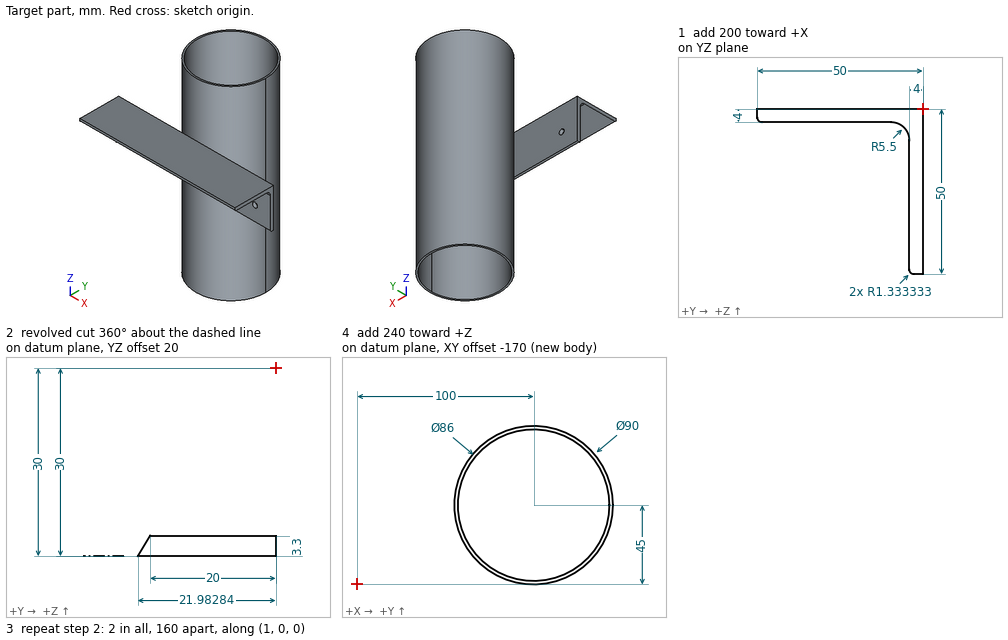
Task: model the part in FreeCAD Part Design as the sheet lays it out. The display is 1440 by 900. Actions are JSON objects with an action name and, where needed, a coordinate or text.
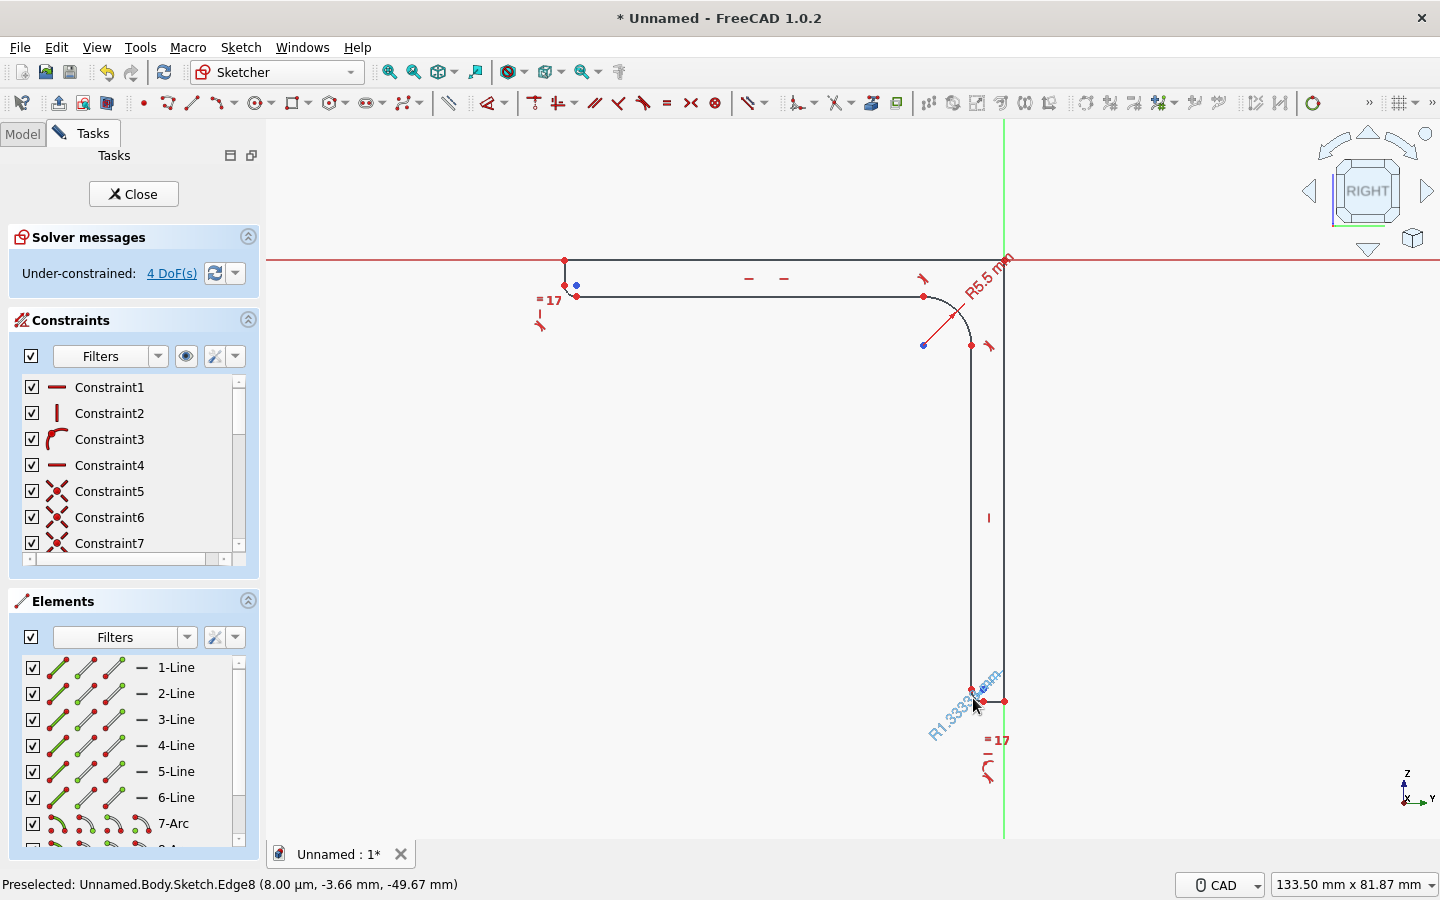
{"action": "left_click", "coordinate": [1004, 569]}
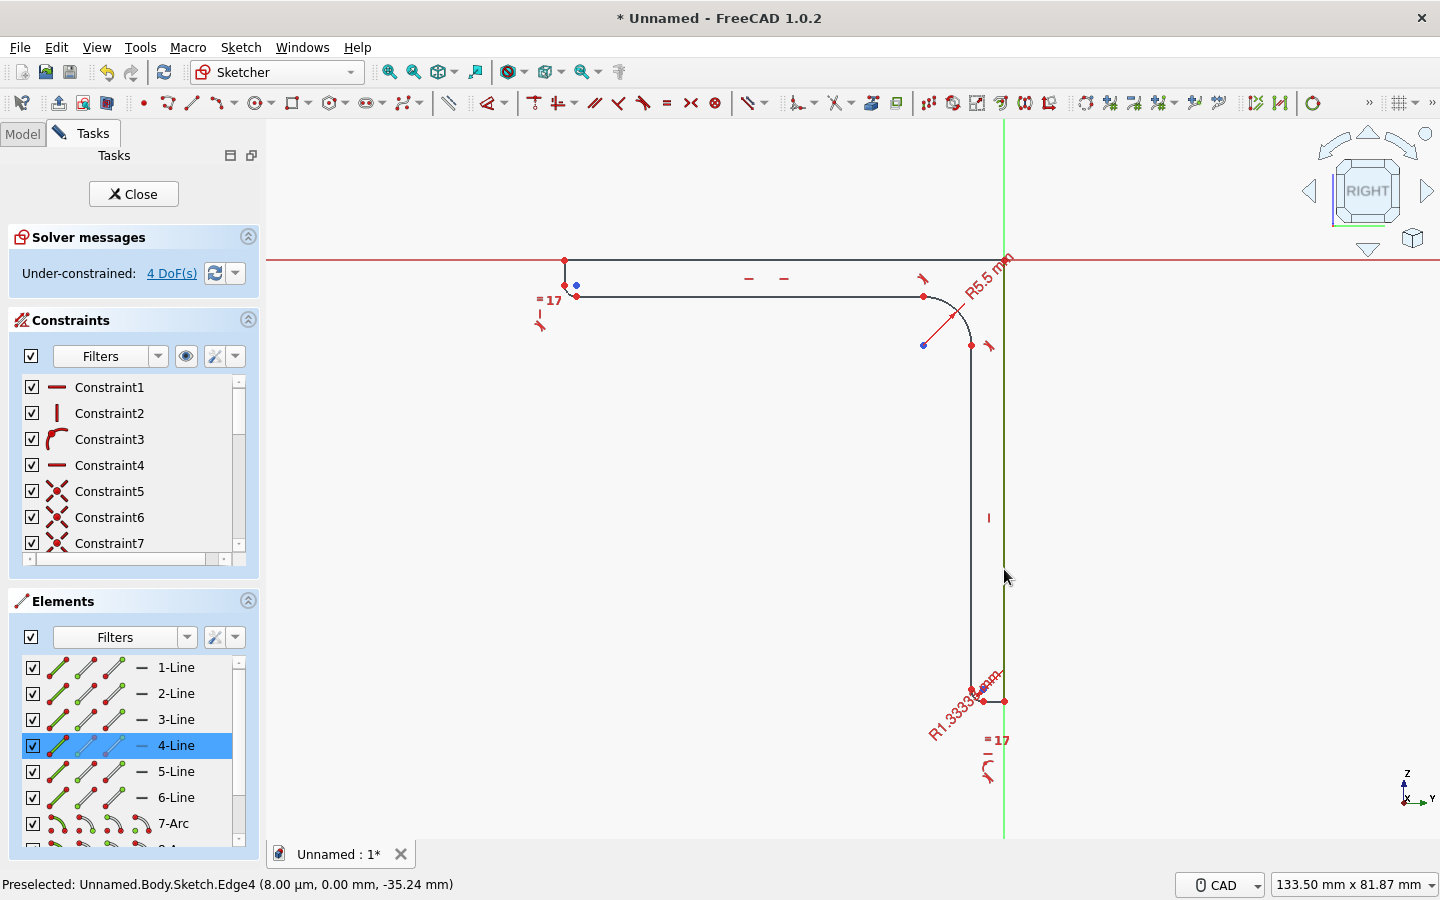
{"action": "key", "text": "i"}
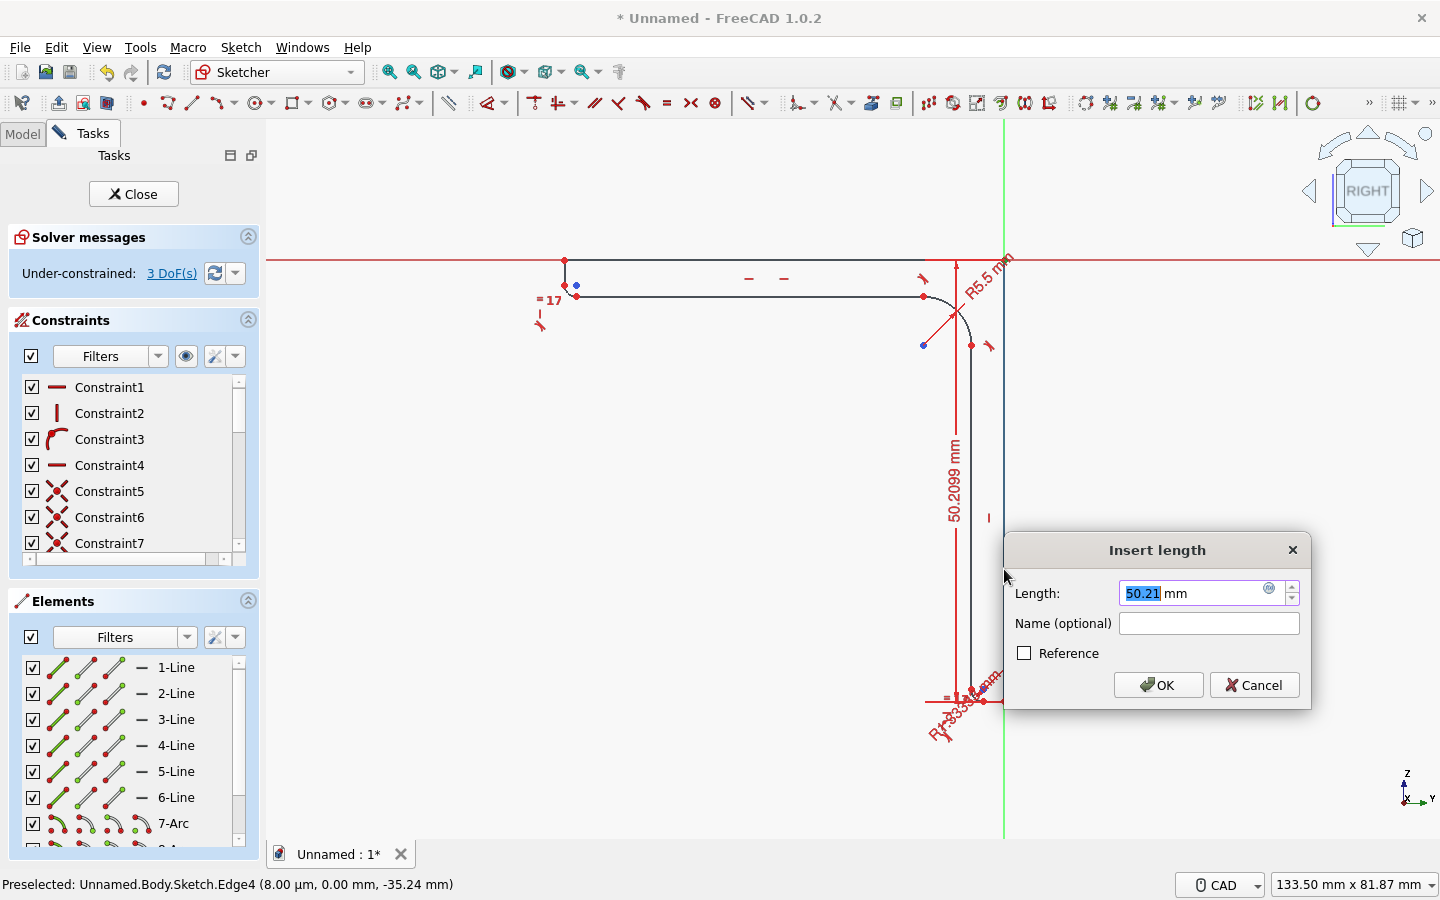
{"action": "type", "text": "50"}
{"action": "key", "text": "Return"}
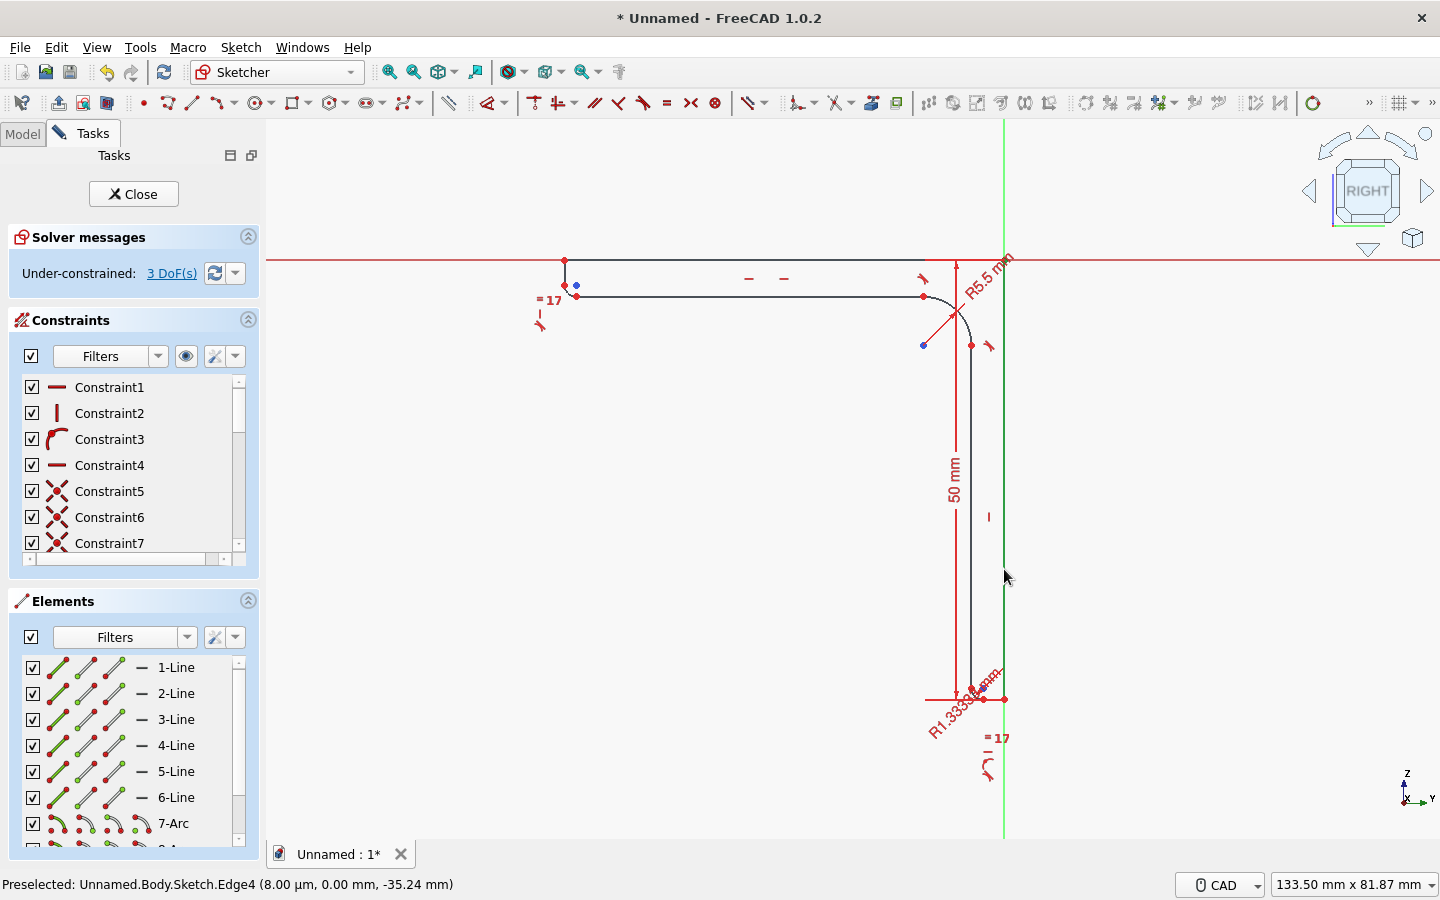
{"action": "left_click", "coordinate": [873, 260]}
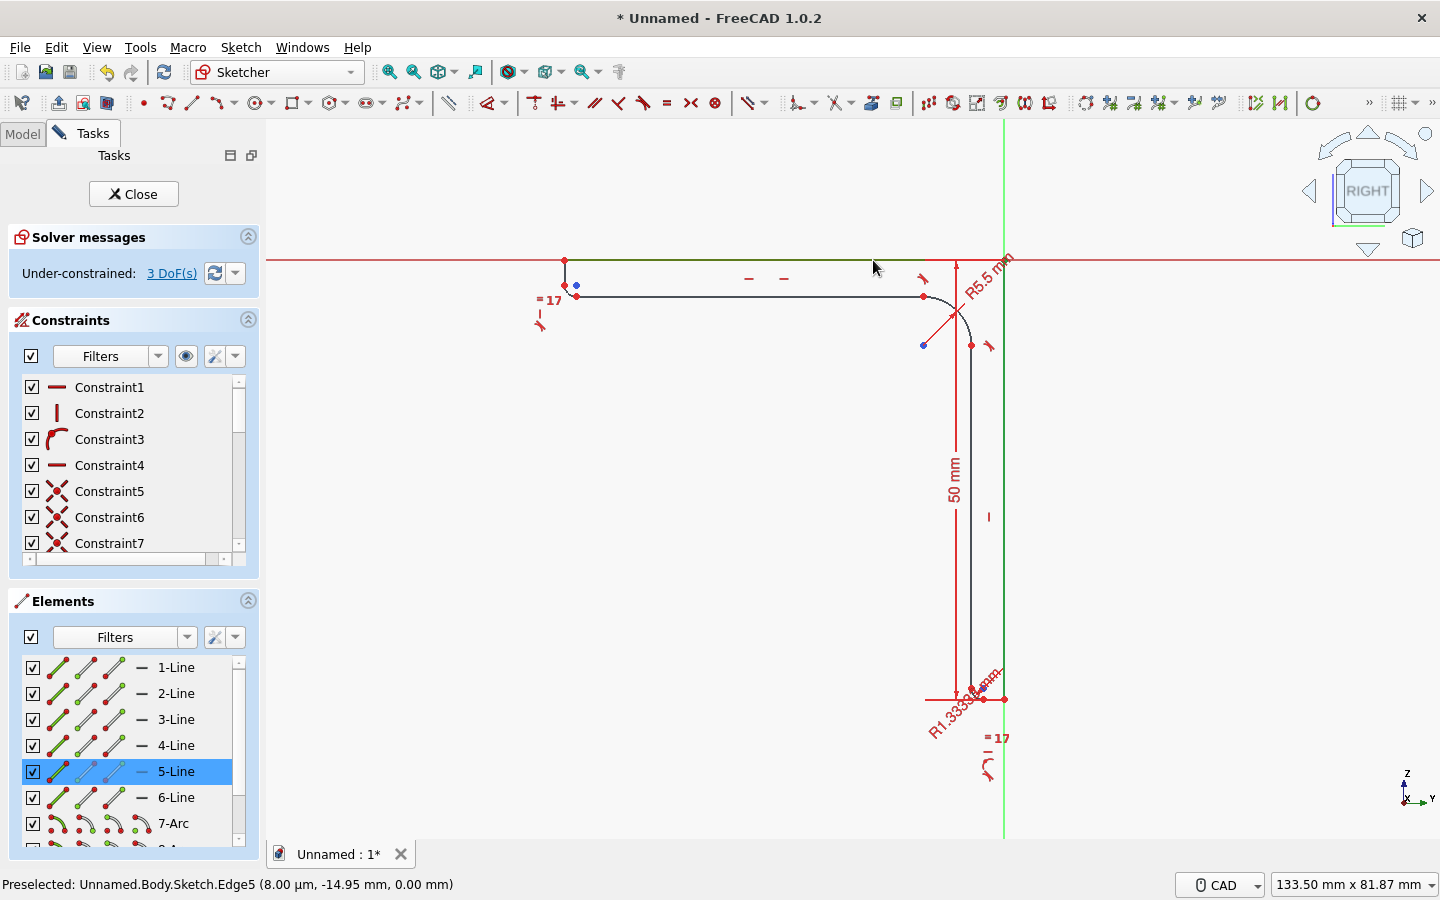
{"action": "key", "text": "l"}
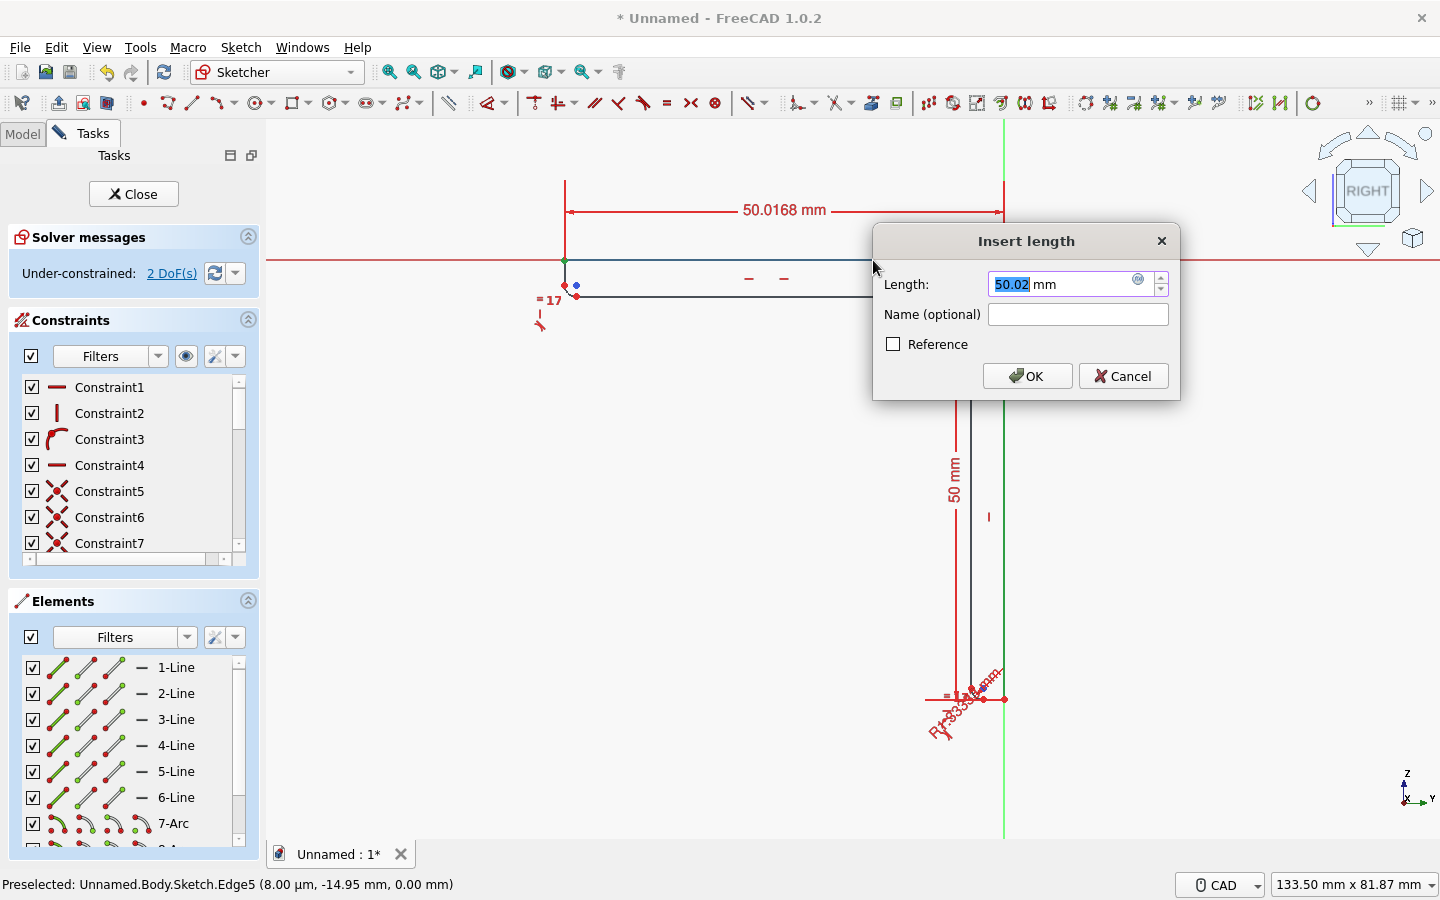
{"action": "type", "text": "50"}
{"action": "key", "text": "Return"}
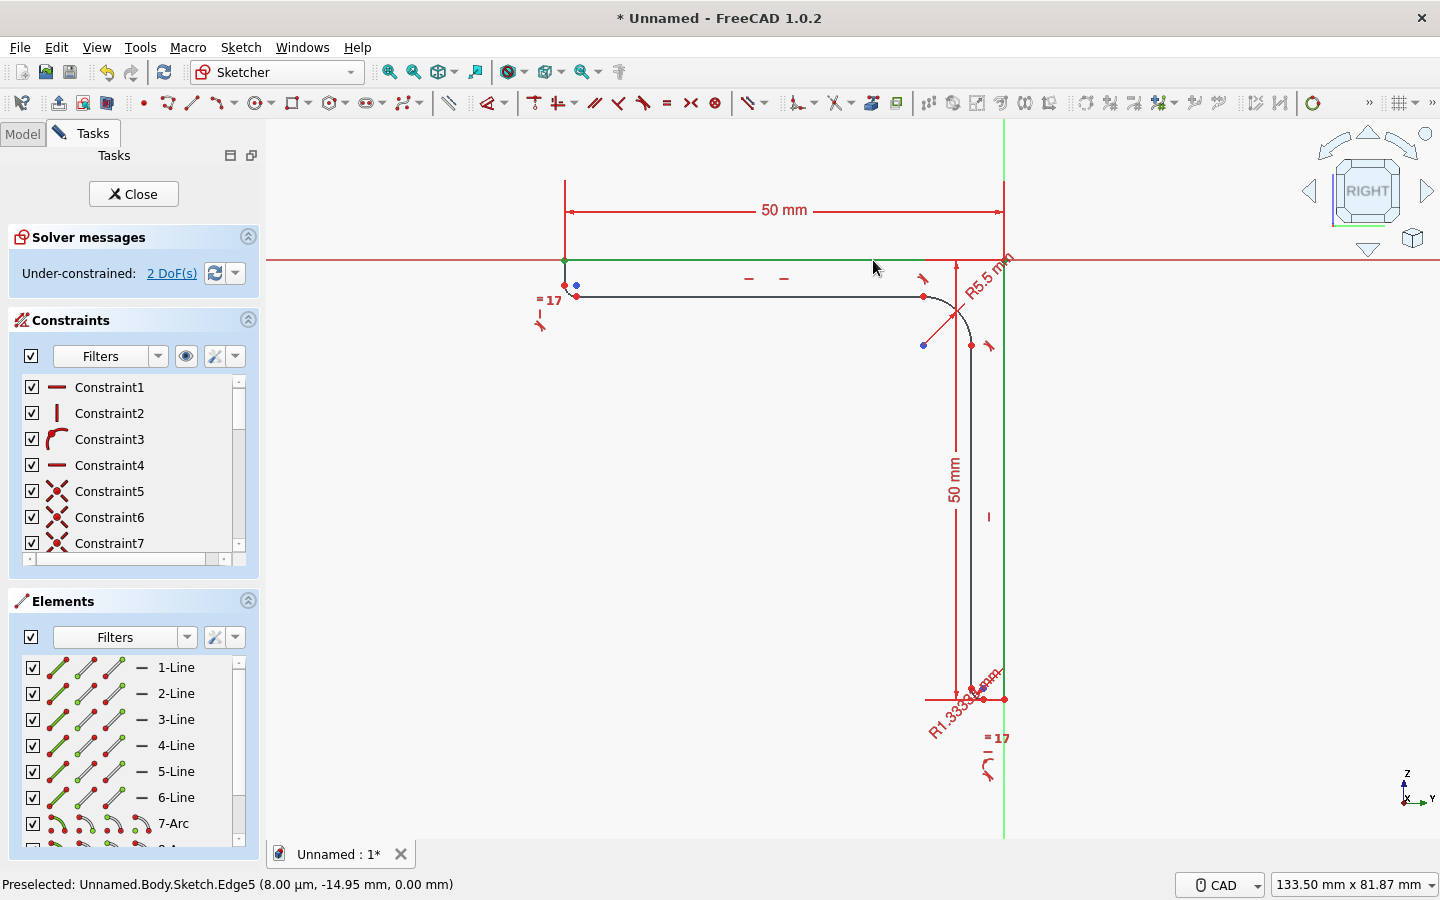
{"action": "left_click", "coordinate": [577, 297]}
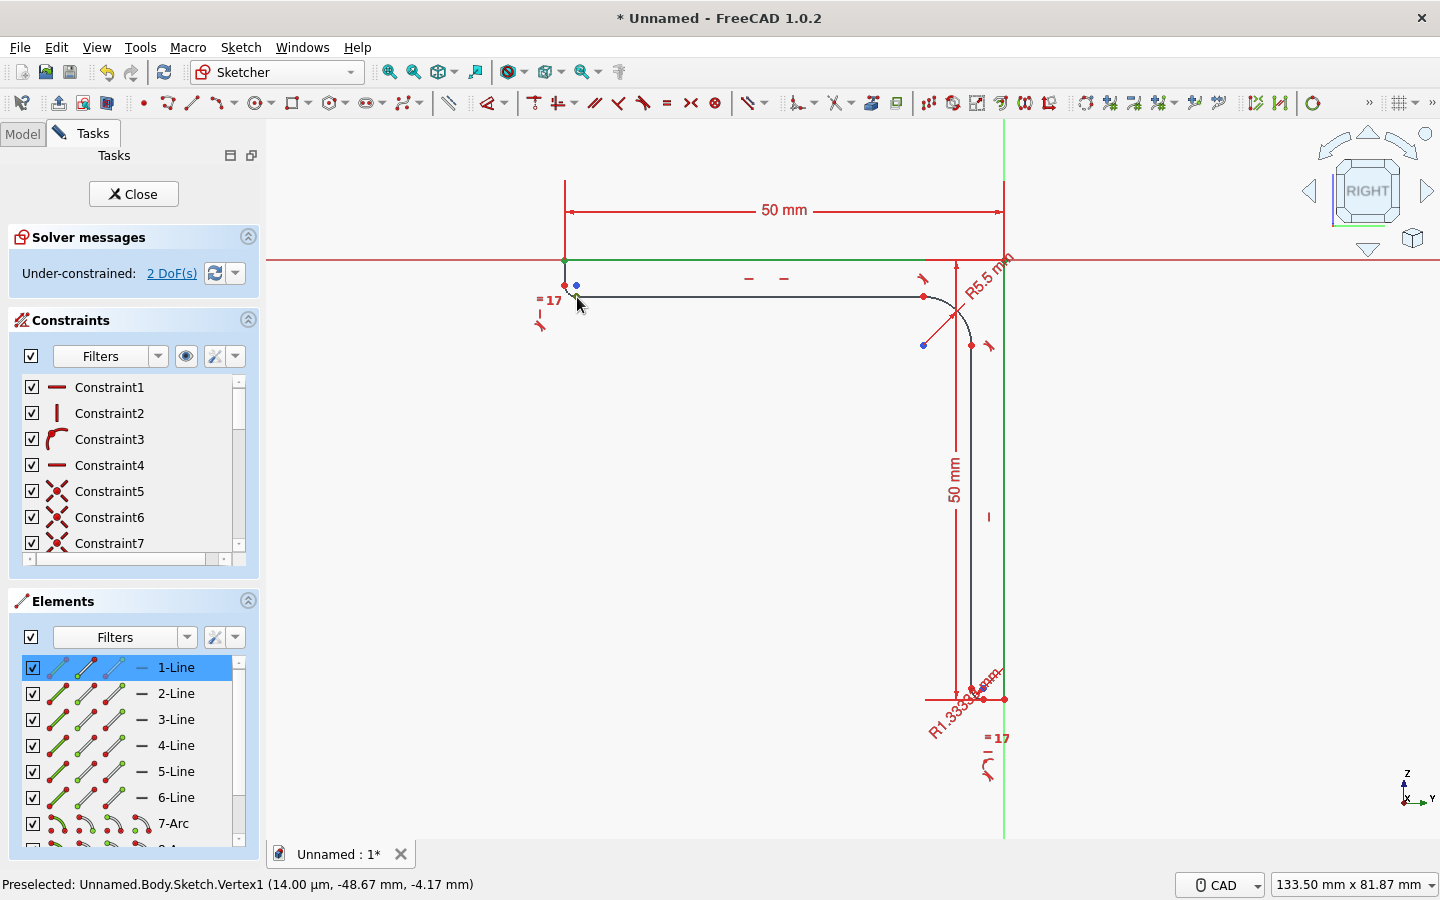
{"action": "left_click", "coordinate": [506, 104]}